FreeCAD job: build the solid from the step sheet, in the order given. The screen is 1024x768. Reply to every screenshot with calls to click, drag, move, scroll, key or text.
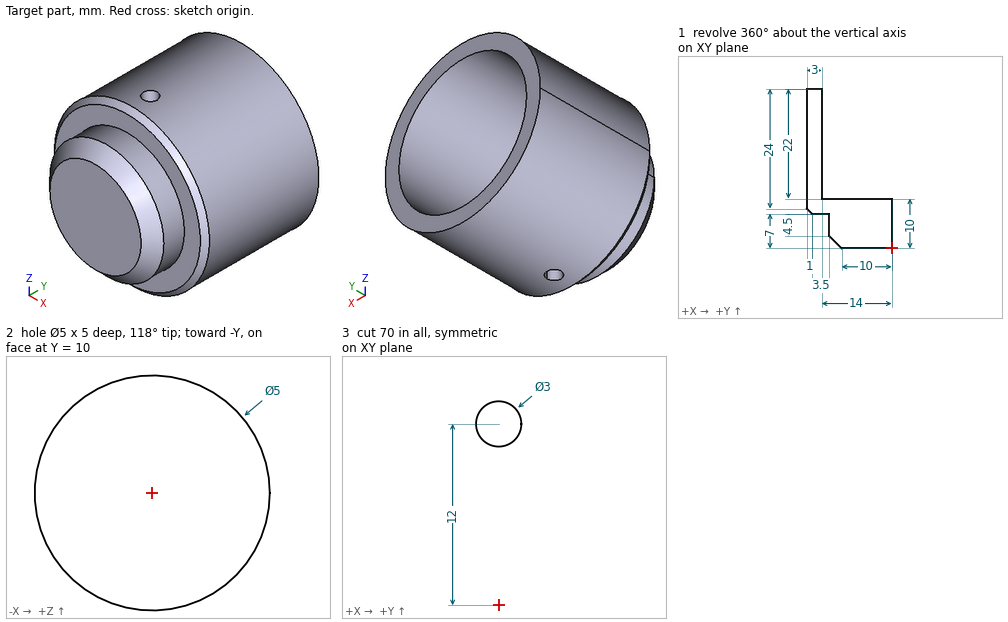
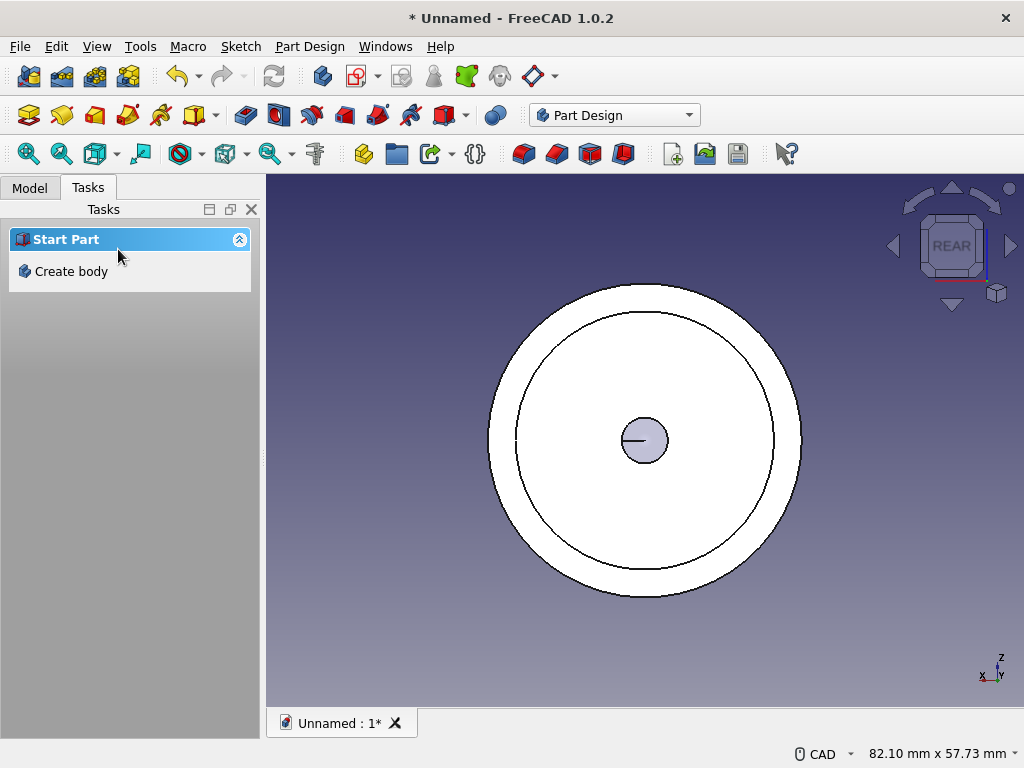
key(0)